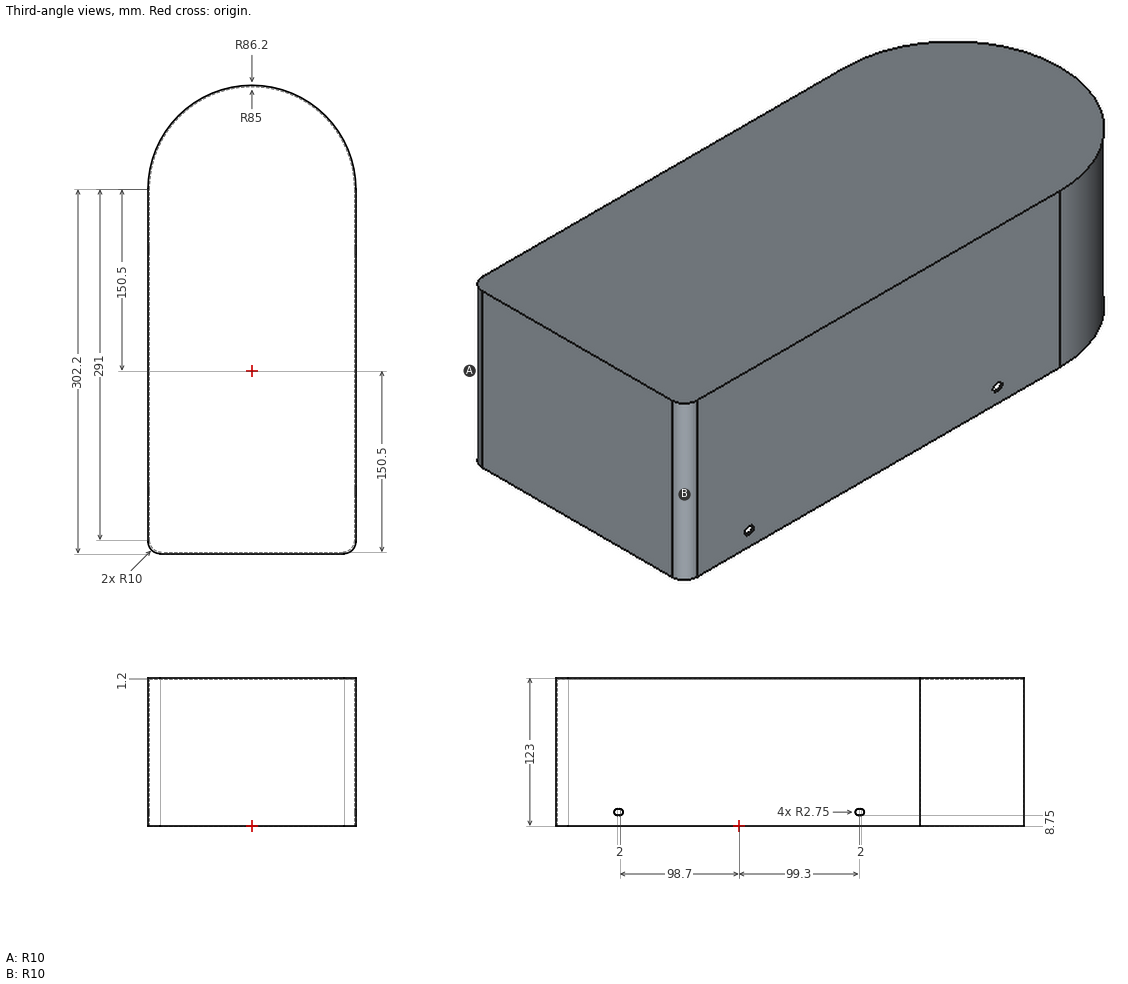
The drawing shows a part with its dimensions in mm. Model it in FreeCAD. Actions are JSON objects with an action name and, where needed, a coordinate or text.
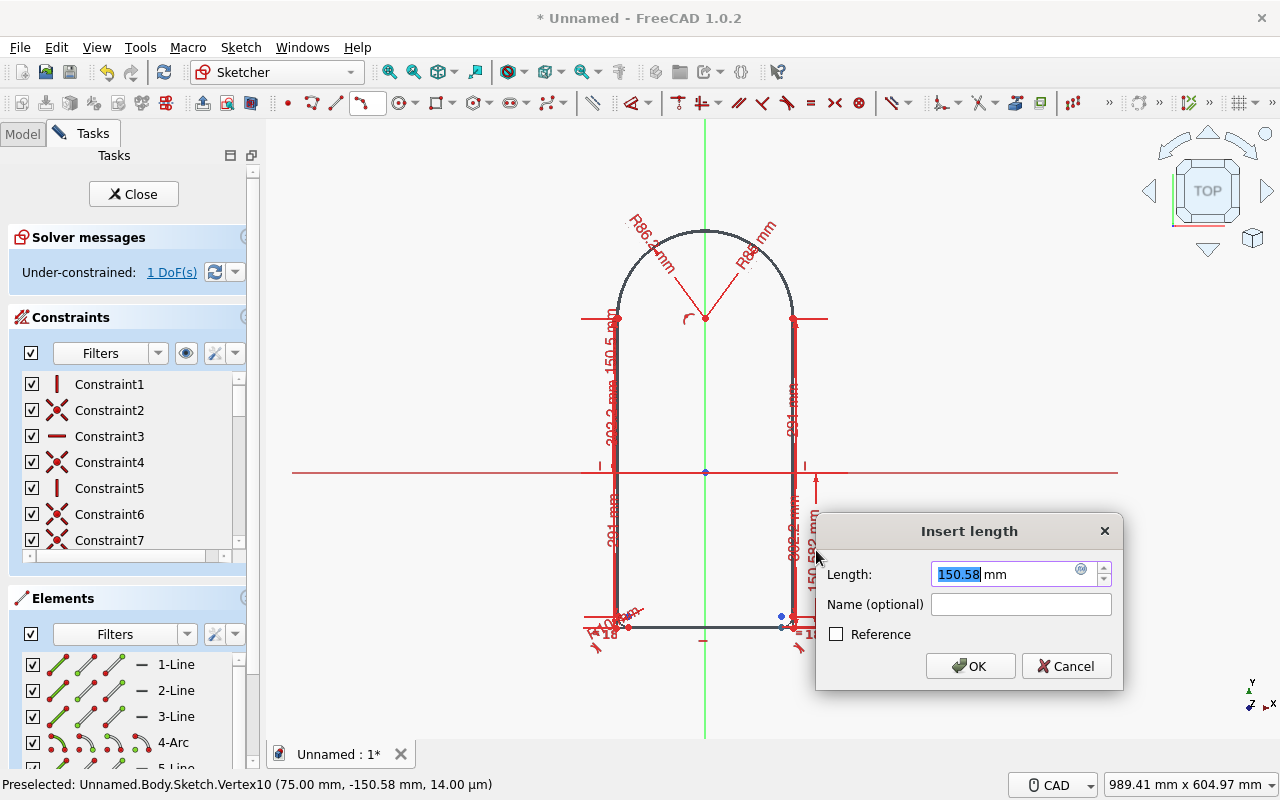
{"action": "type", "text": "150.5"}
{"action": "key", "text": "Return"}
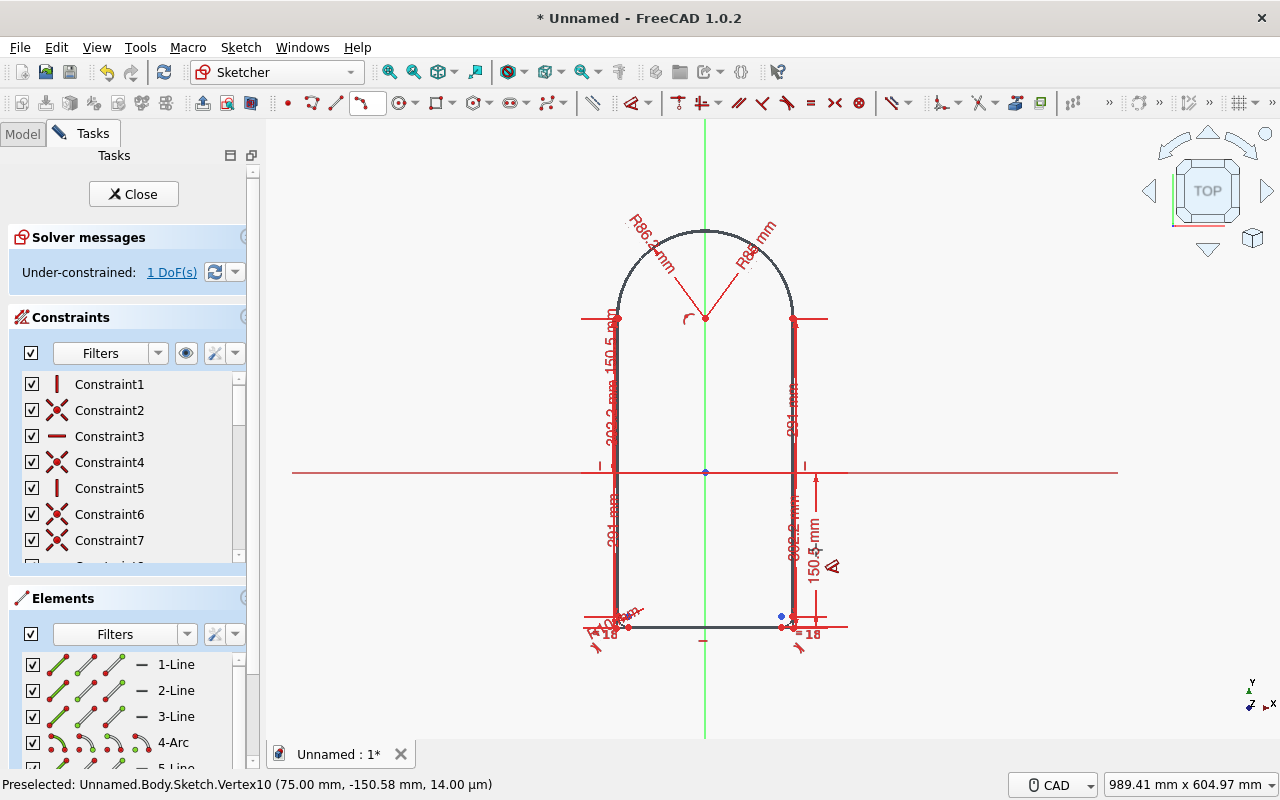
{"action": "left_click", "coordinate": [705, 319]}
{"action": "left_click", "coordinate": [739, 360]}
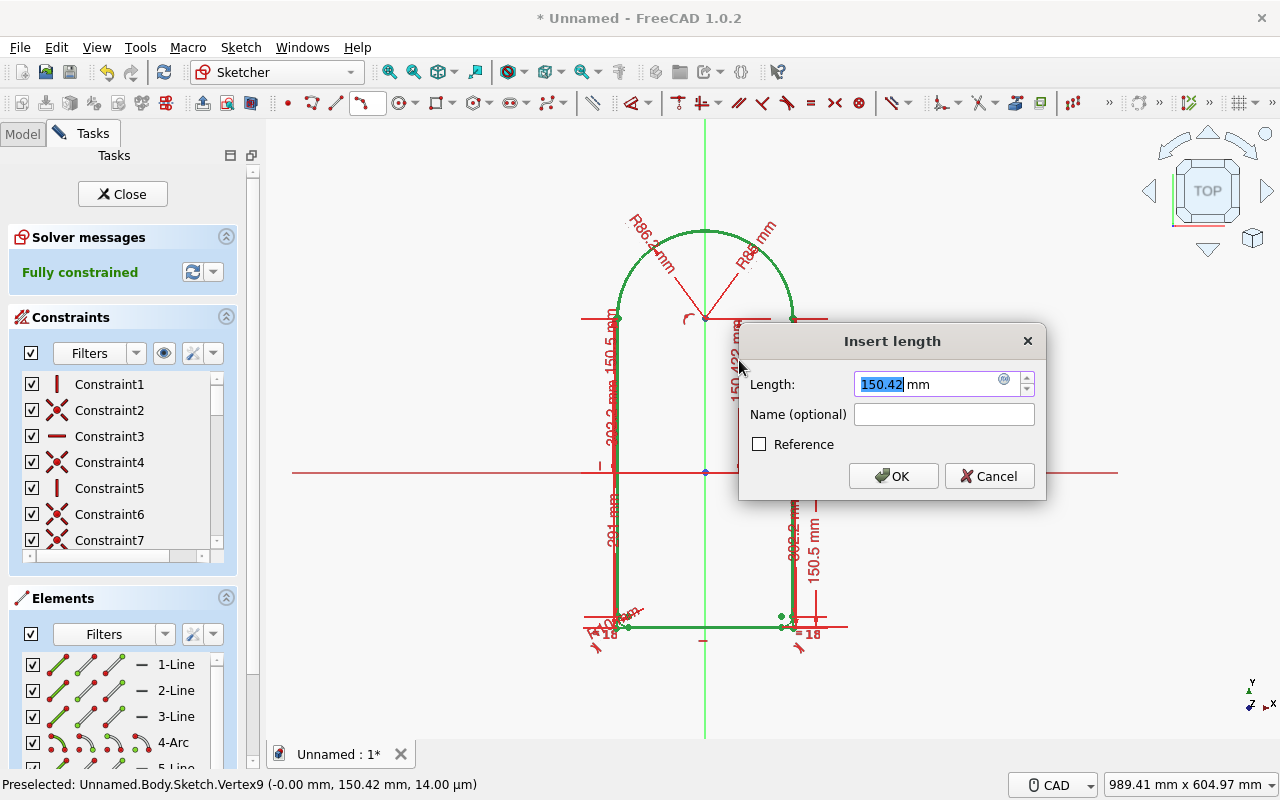
{"action": "type", "text": "150.5"}
{"action": "key", "text": "Return"}
{"action": "key", "text": "Escape"}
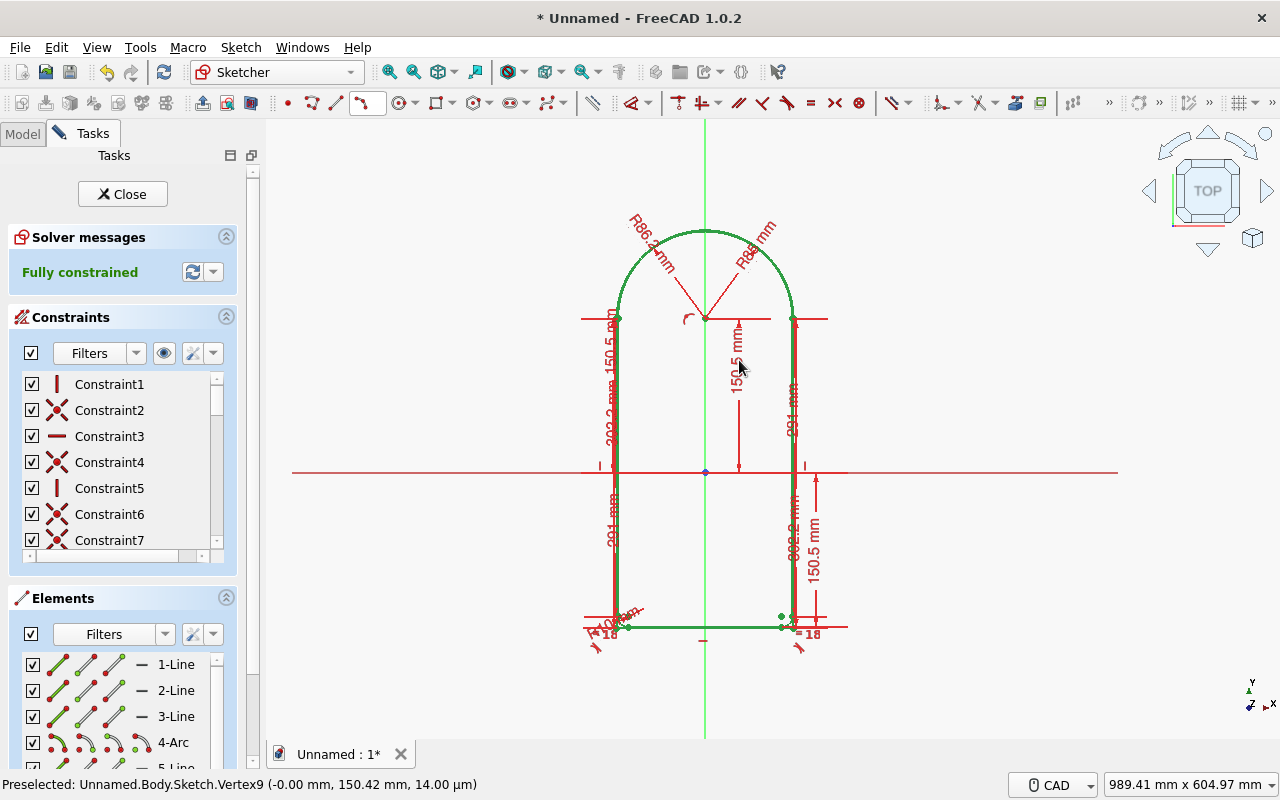
{"action": "left_click", "coordinate": [123, 194]}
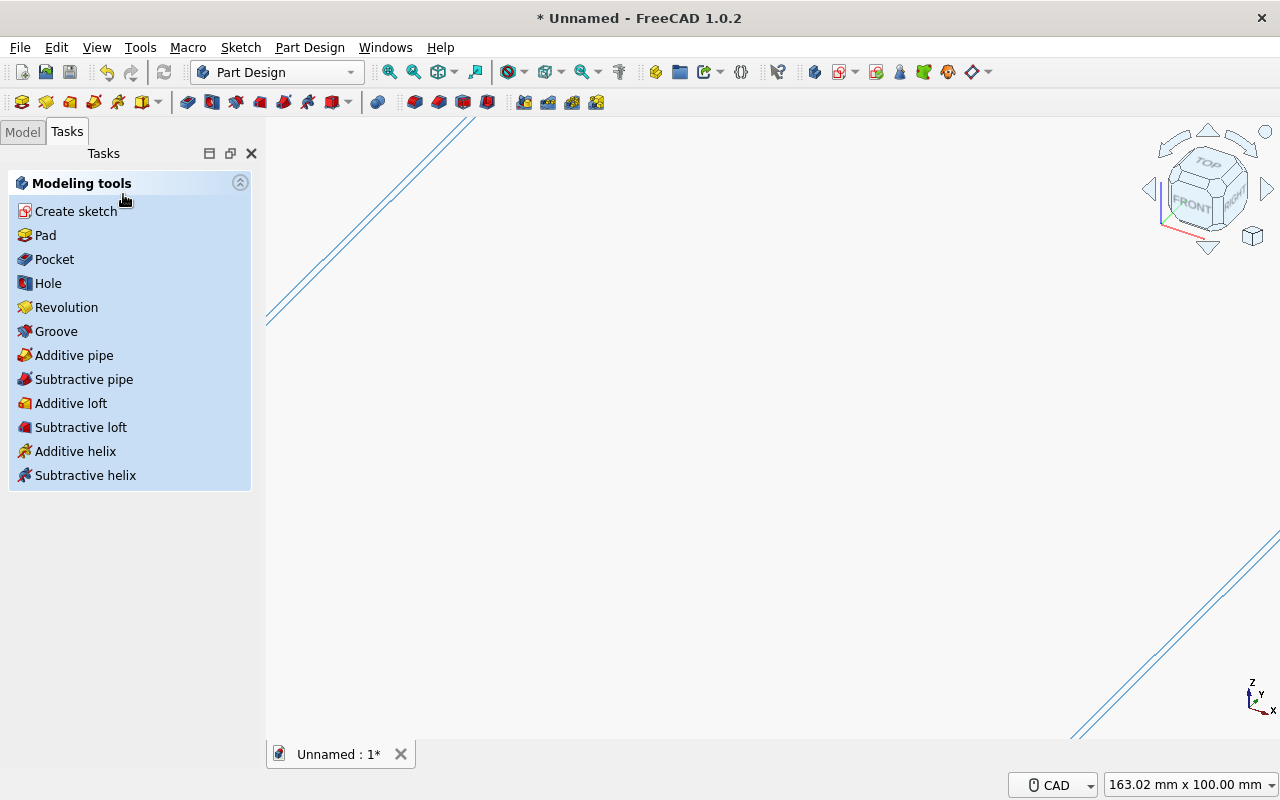
{"action": "left_click", "coordinate": [22, 102]}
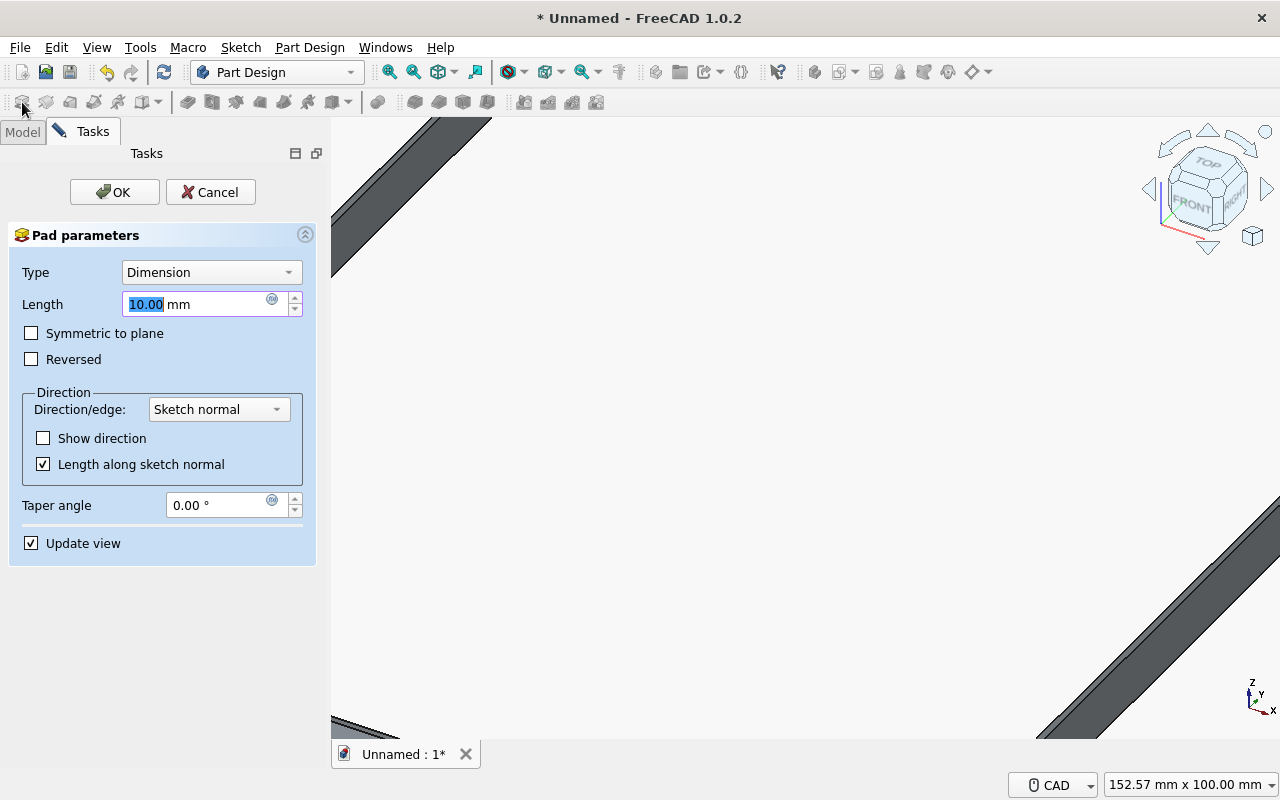
{"action": "type", "text": "123"}
{"action": "key", "text": "Tab"}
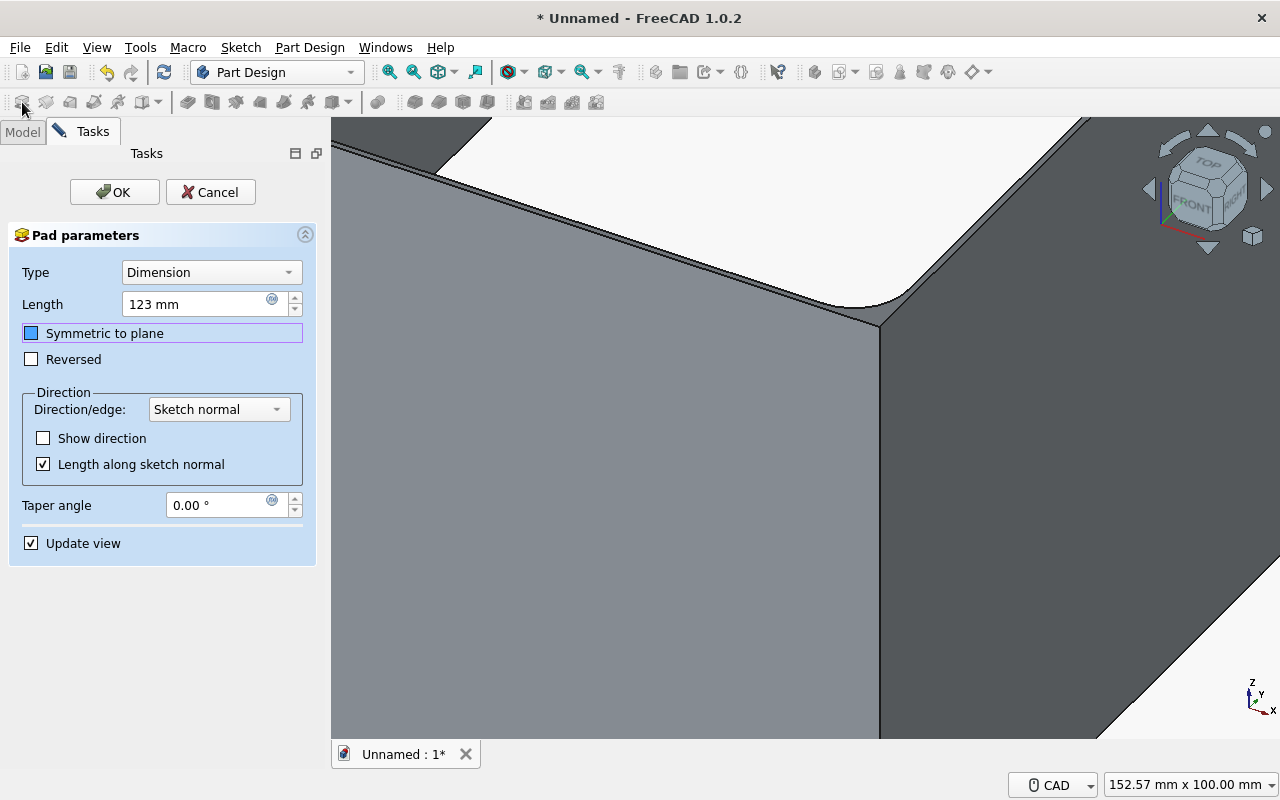
{"action": "left_click", "coordinate": [115, 192]}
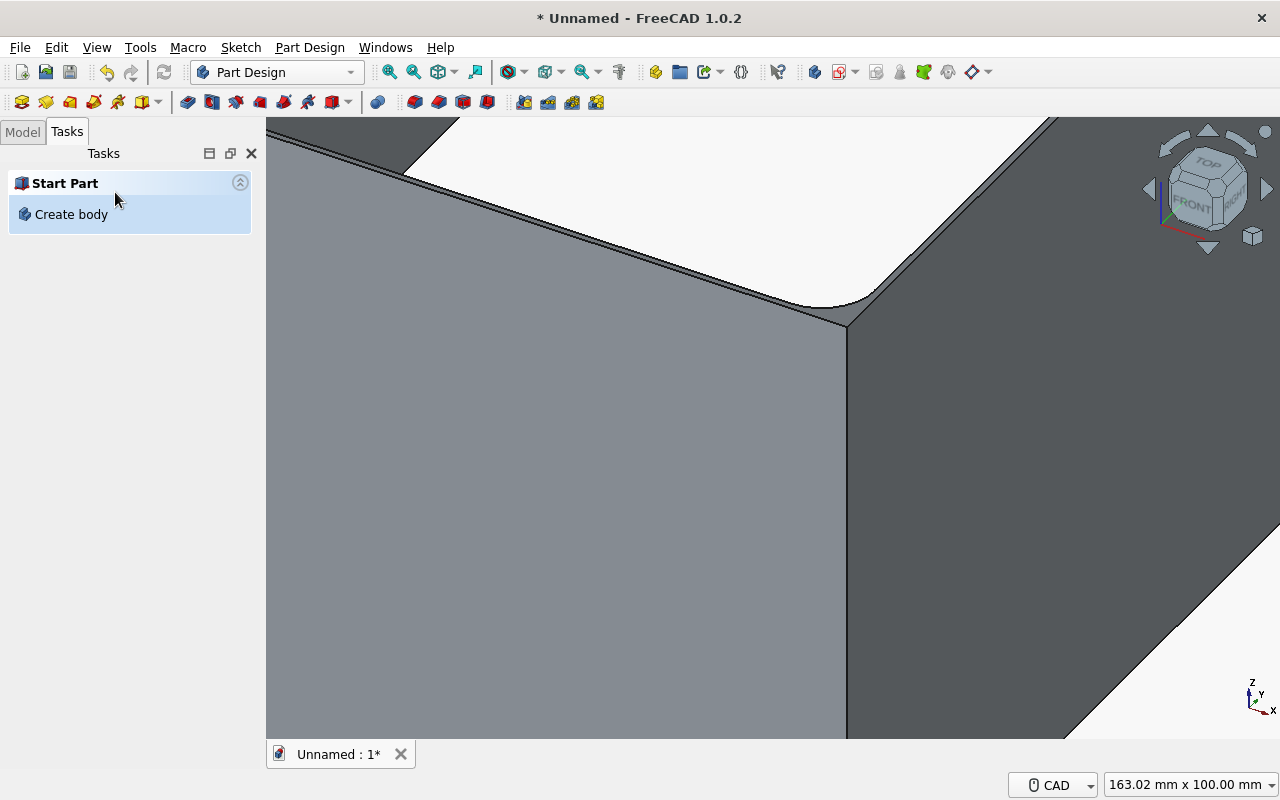
{"action": "left_click", "coordinate": [390, 72]}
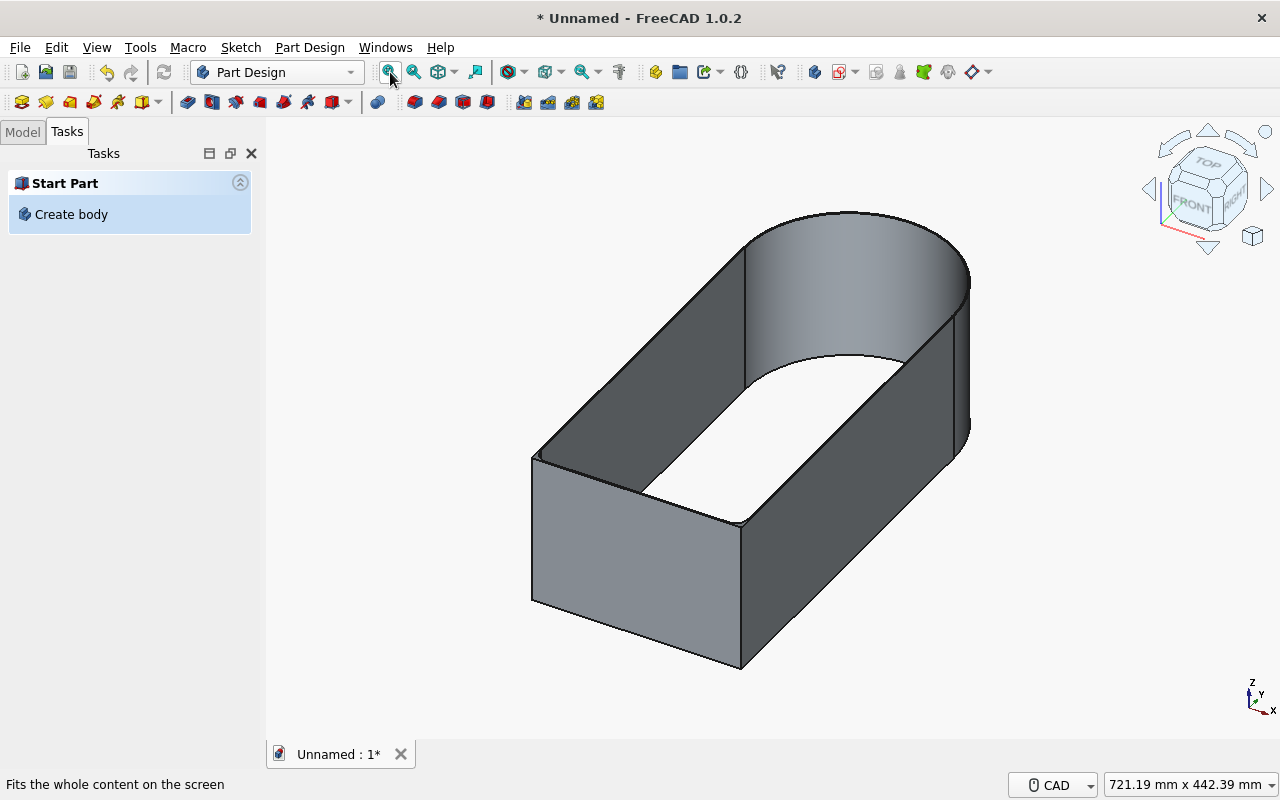
{"action": "left_click", "coordinate": [23, 131]}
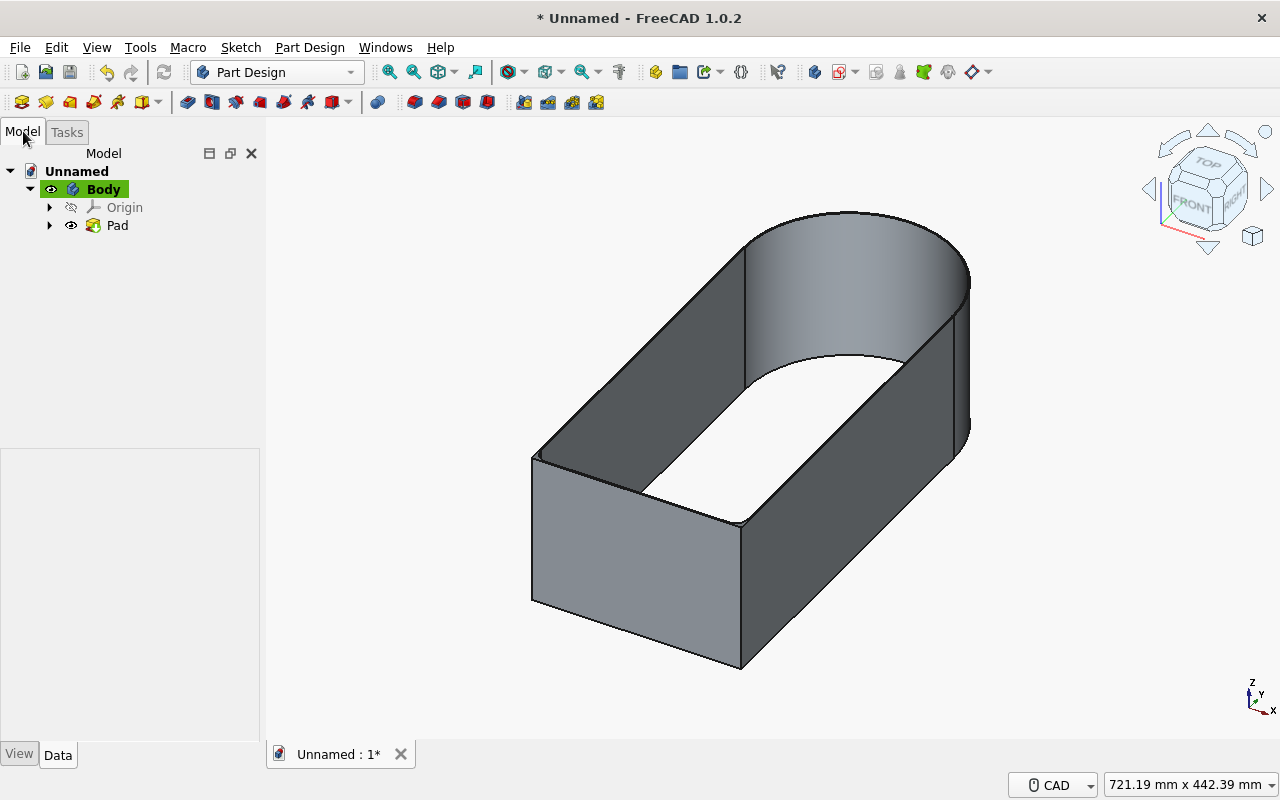
{"action": "left_click", "coordinate": [50, 207]}